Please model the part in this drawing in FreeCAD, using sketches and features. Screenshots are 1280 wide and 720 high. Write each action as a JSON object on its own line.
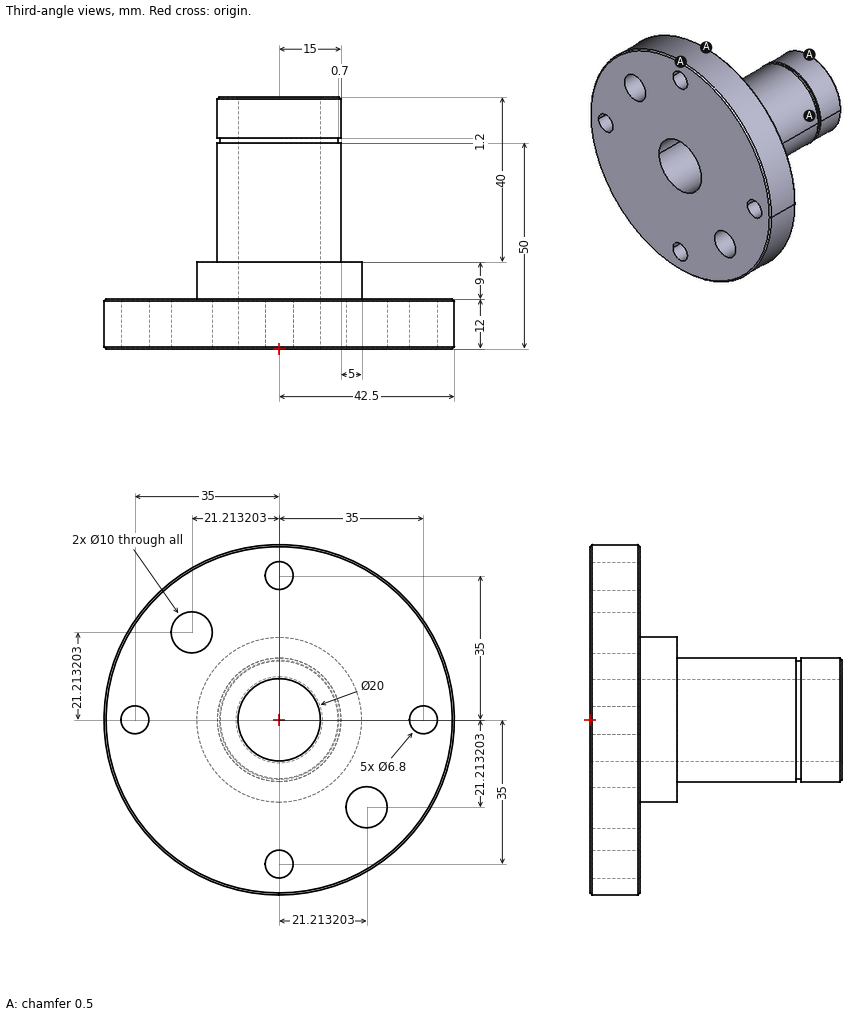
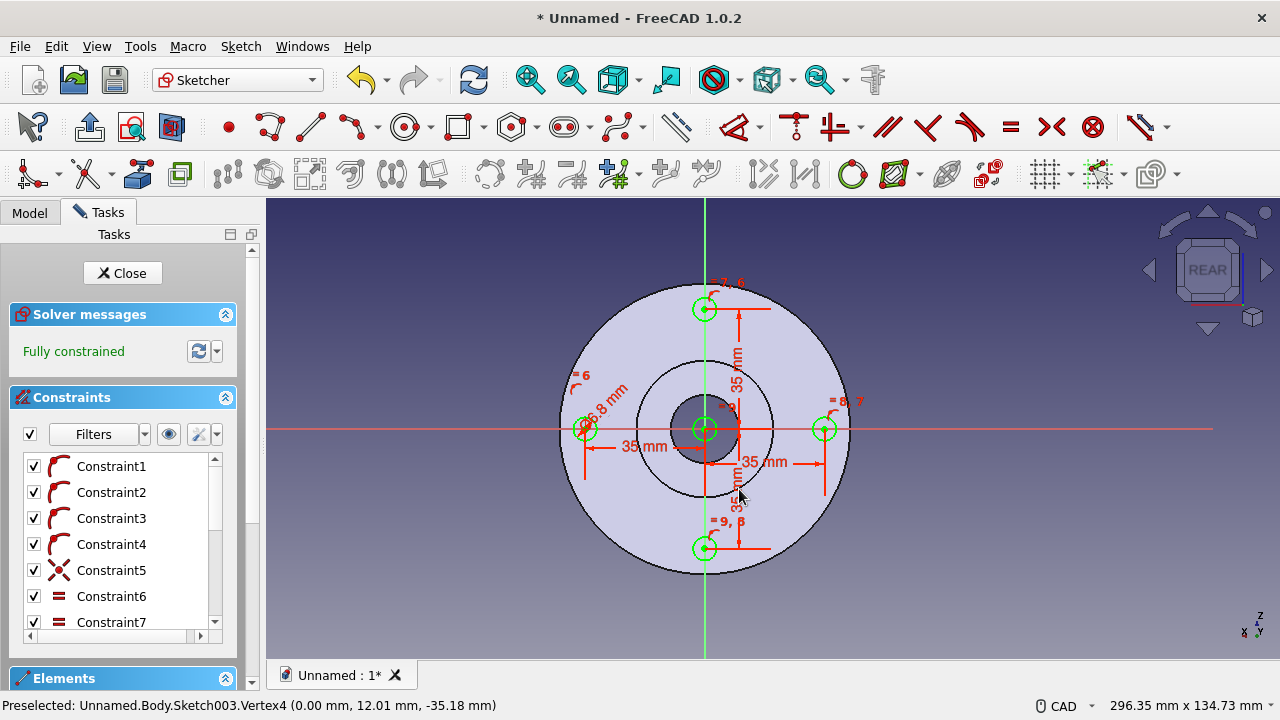
{"action": "left_click", "coordinate": [123, 273]}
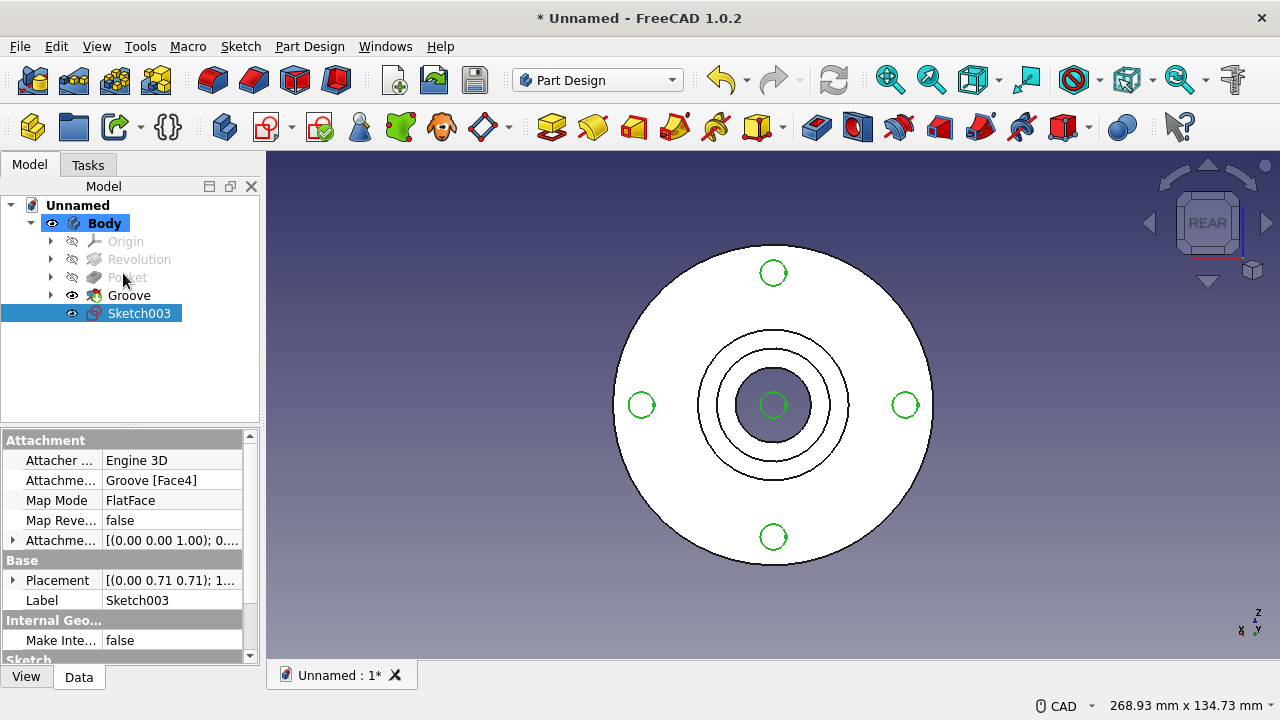
{"action": "left_click", "coordinate": [817, 128]}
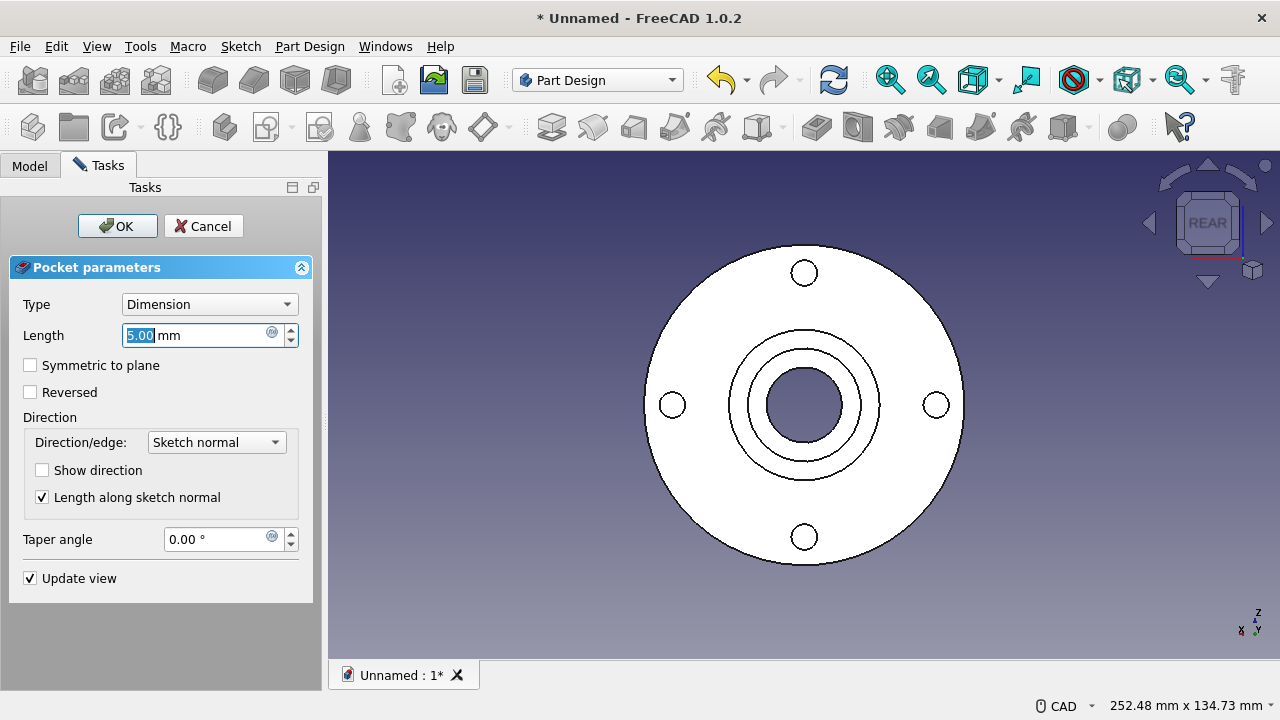
{"action": "left_click", "coordinate": [210, 304]}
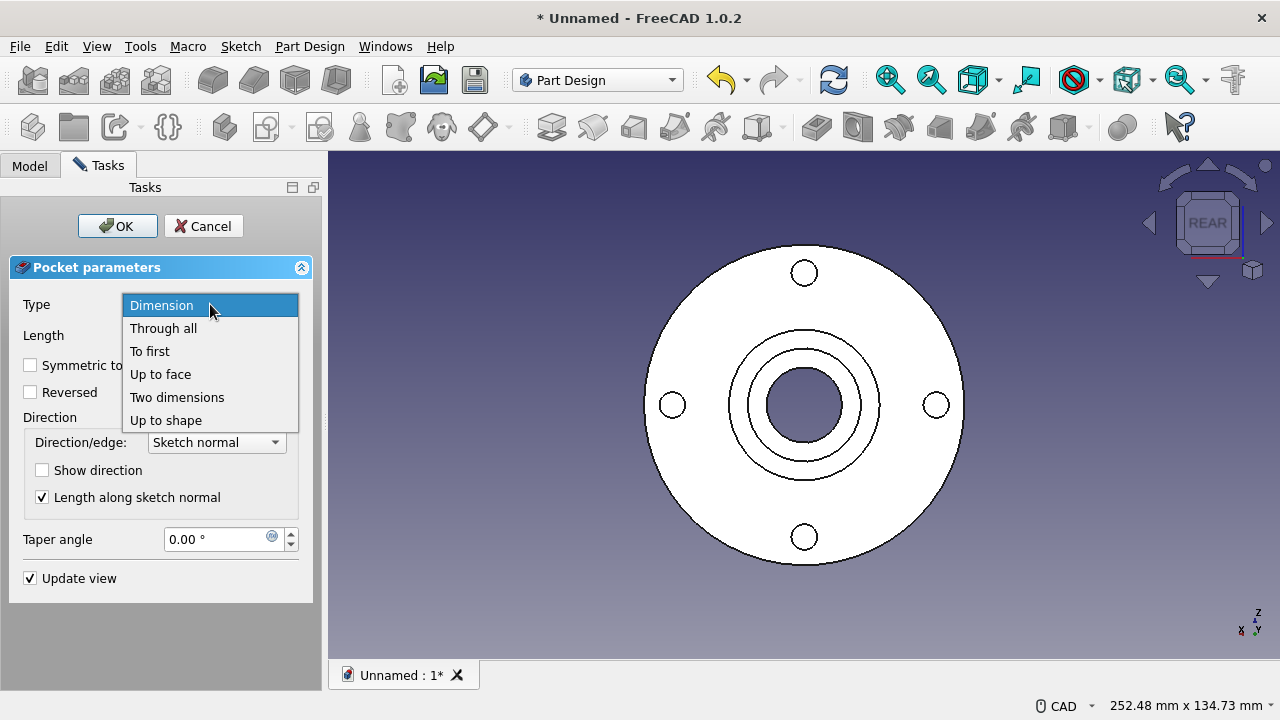
{"action": "left_click", "coordinate": [208, 328]}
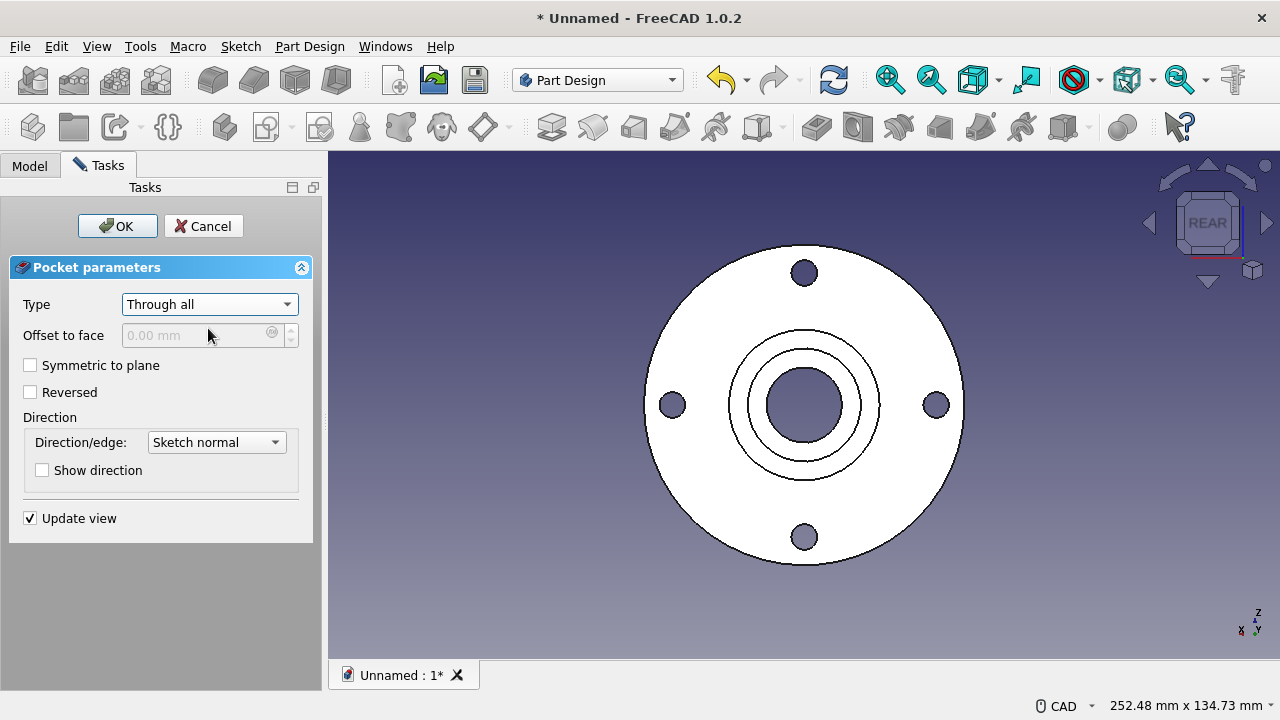
{"action": "left_click", "coordinate": [118, 226]}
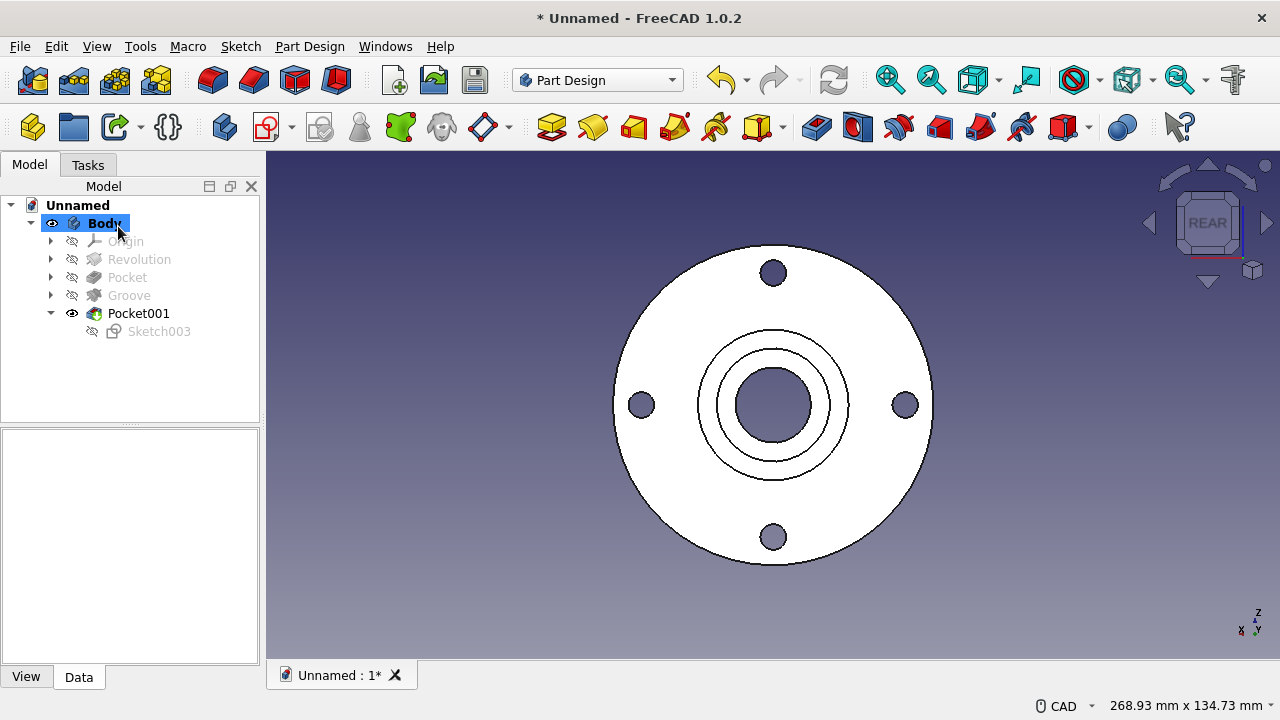
{"action": "left_click", "coordinate": [865, 496]}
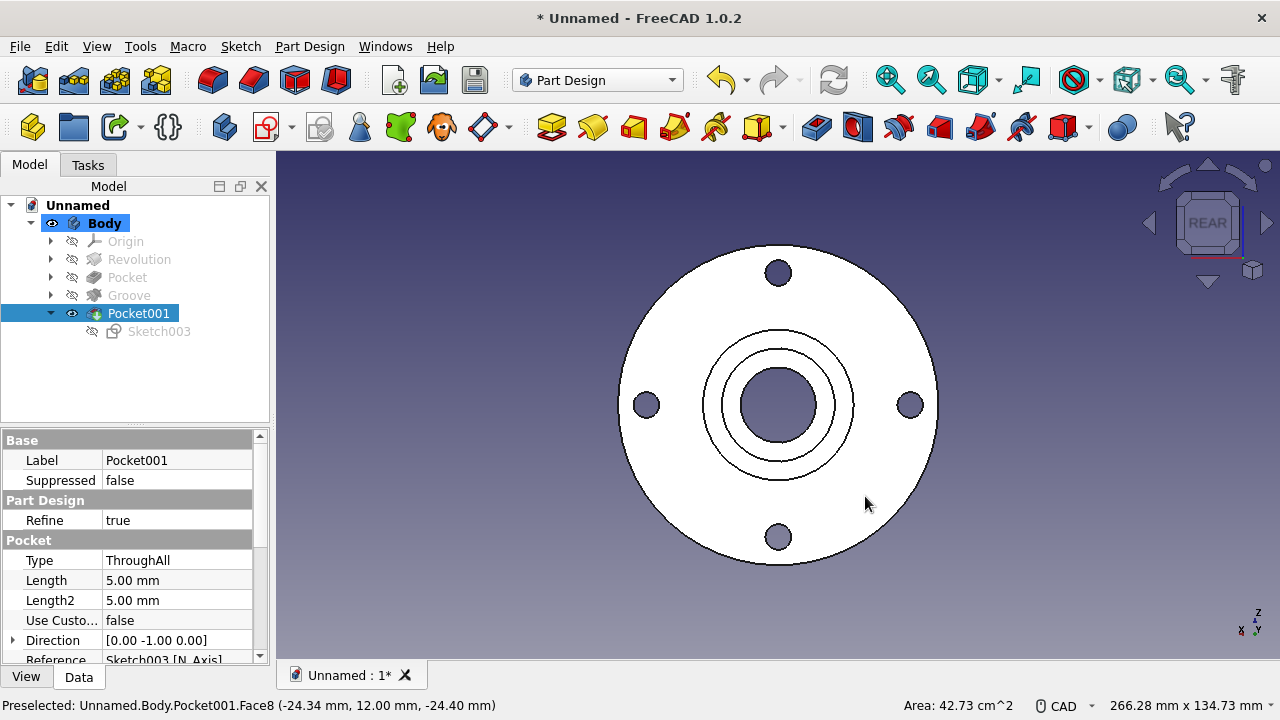
{"action": "left_click", "coordinate": [266, 128]}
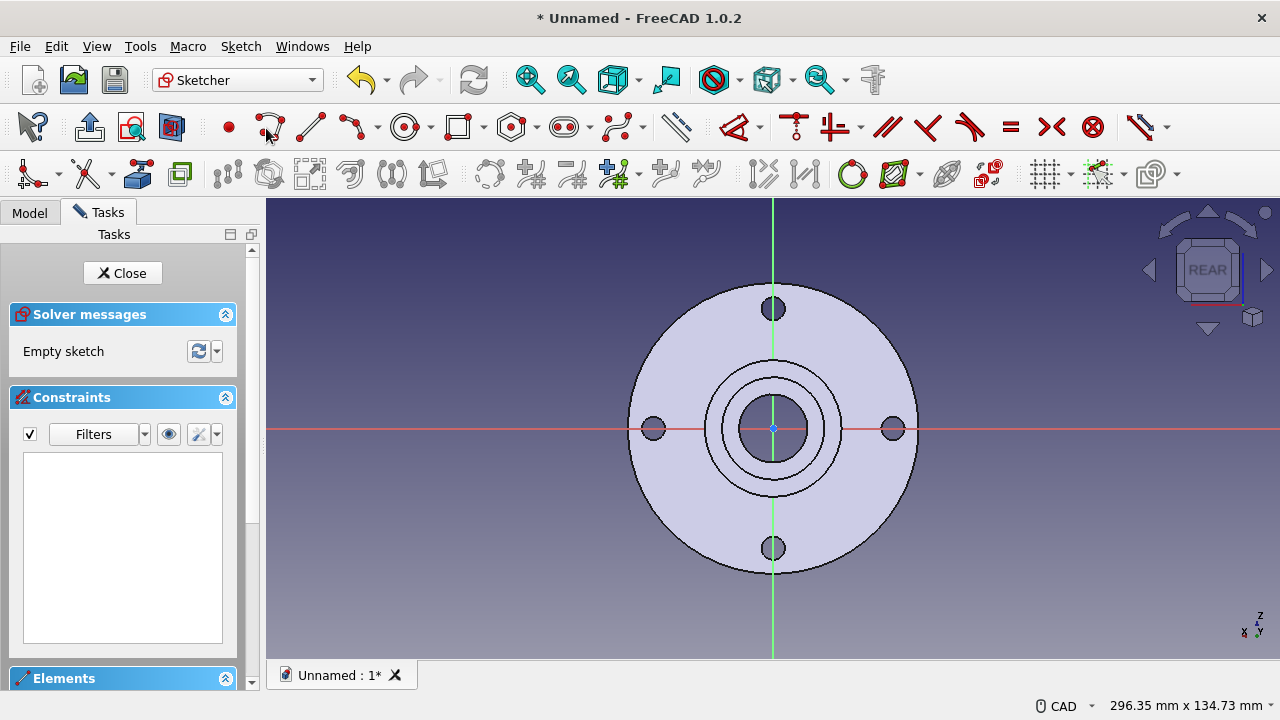
{"action": "scroll", "coordinate": [913, 429], "scroll_direction": "up", "scroll_amount": 2}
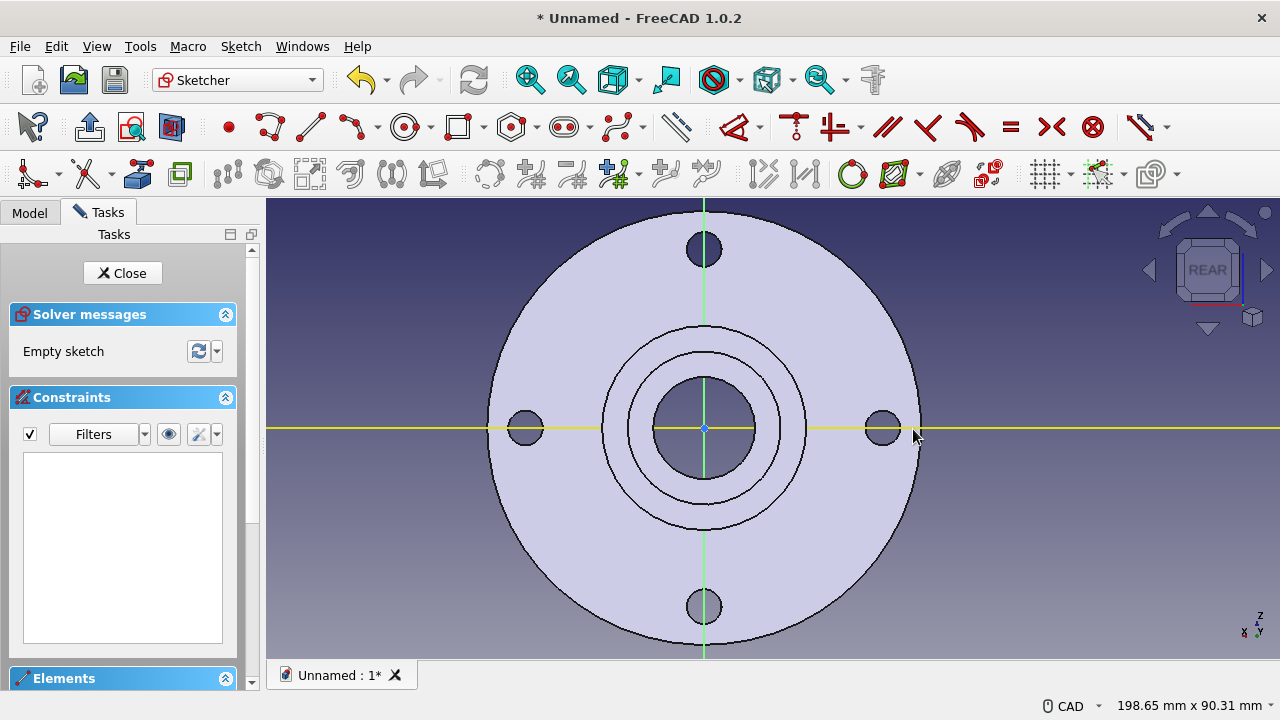
{"action": "left_click", "coordinate": [404, 128]}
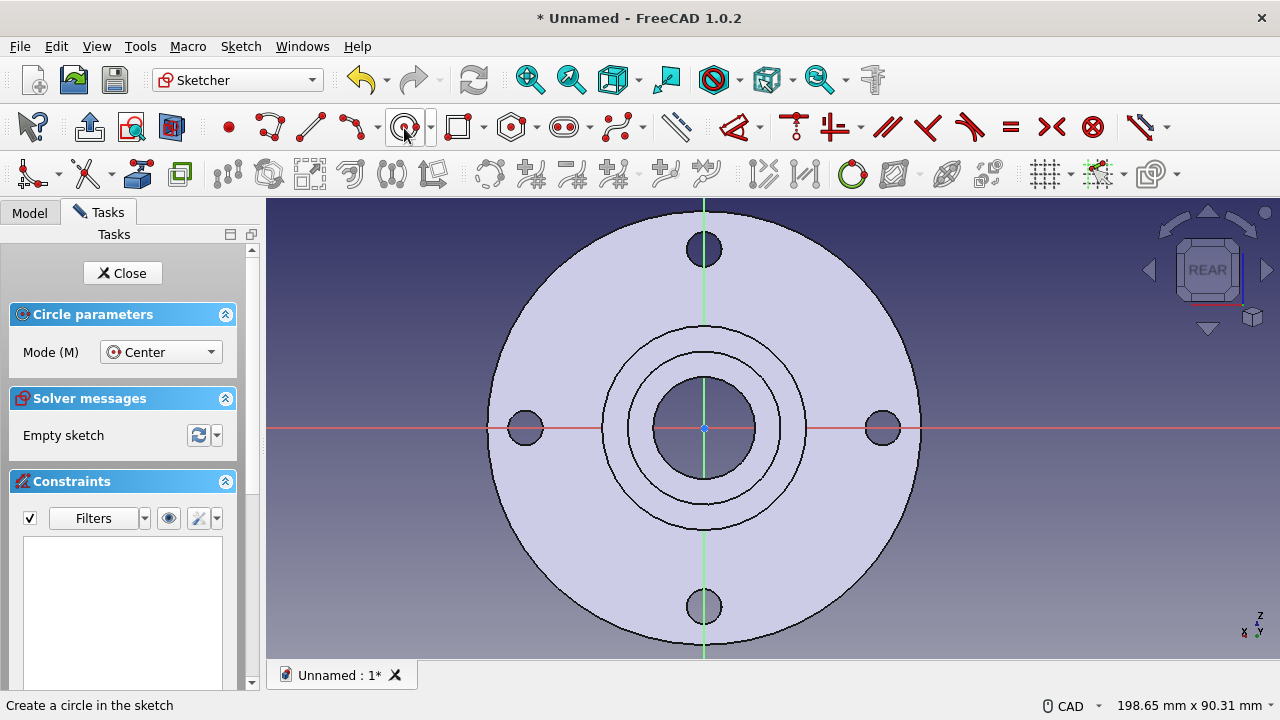
{"action": "left_click", "coordinate": [812, 320]}
{"action": "left_click", "coordinate": [830, 302]}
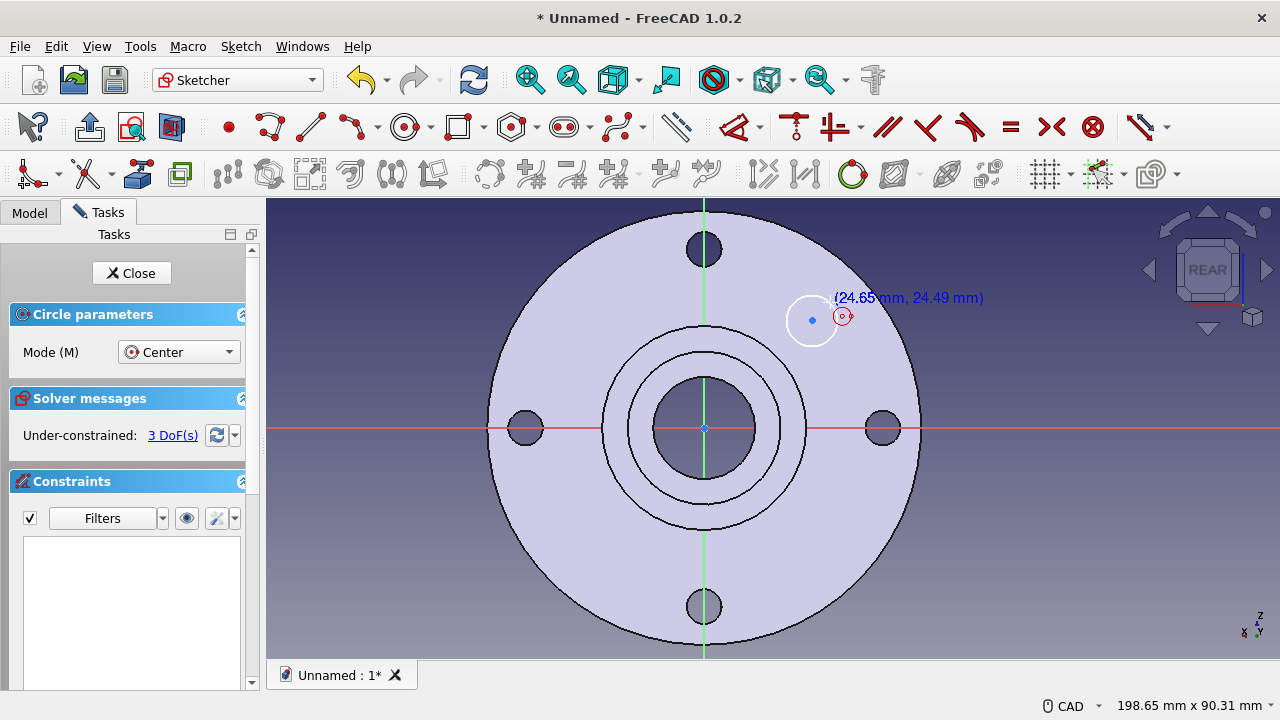
{"action": "left_click", "coordinate": [596, 536]}
{"action": "left_click", "coordinate": [614, 518]}
{"action": "key", "text": "Escape"}